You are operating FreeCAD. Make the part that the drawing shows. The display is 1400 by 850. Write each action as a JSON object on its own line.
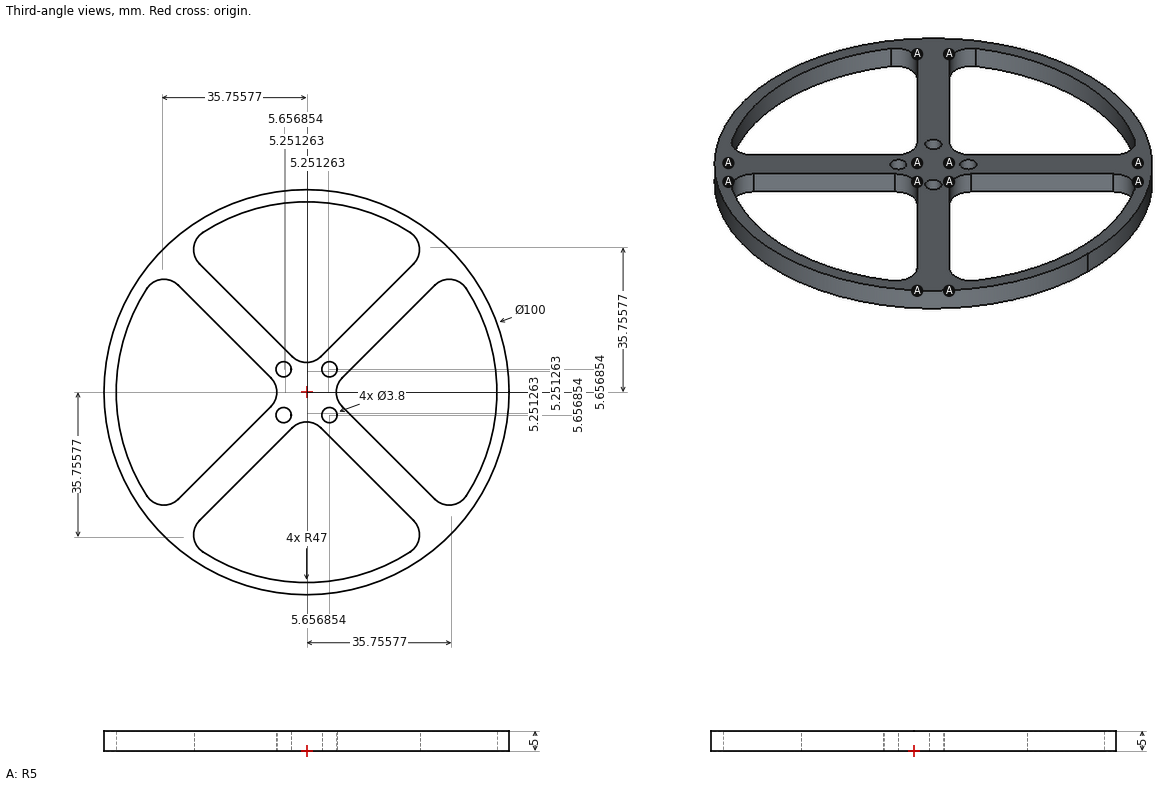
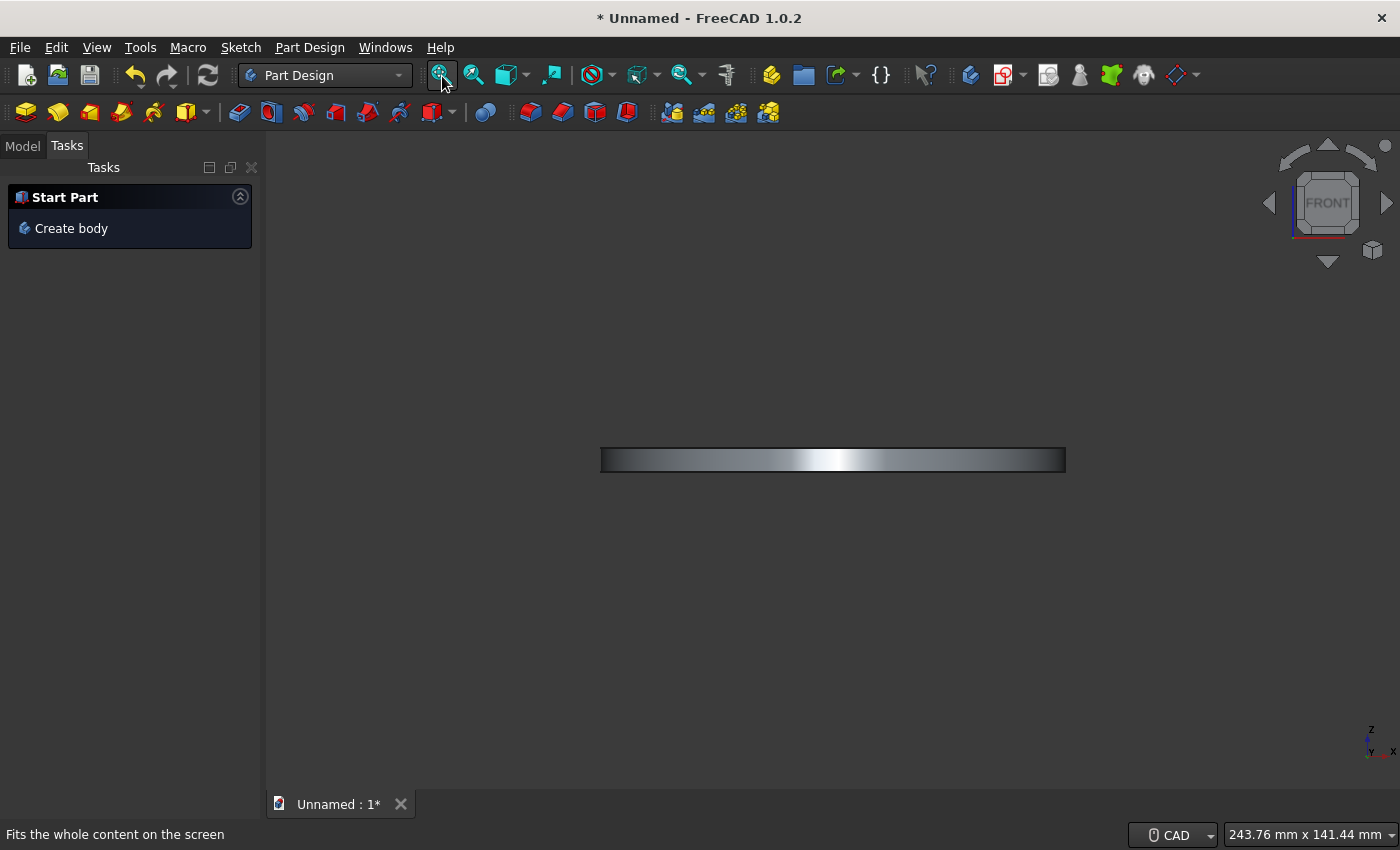
{"action": "left_click", "coordinate": [442, 76]}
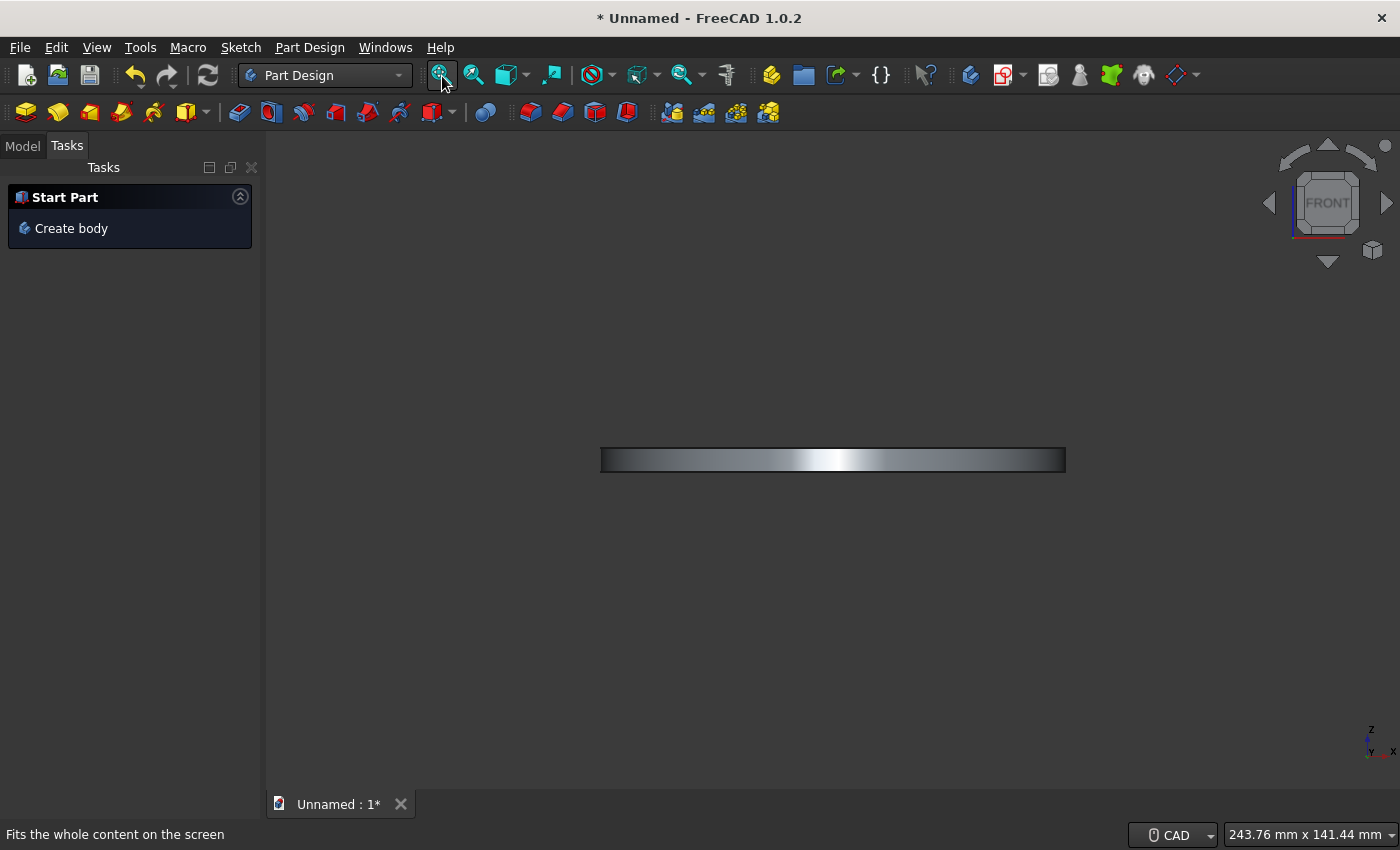
{"action": "key", "text": "3"}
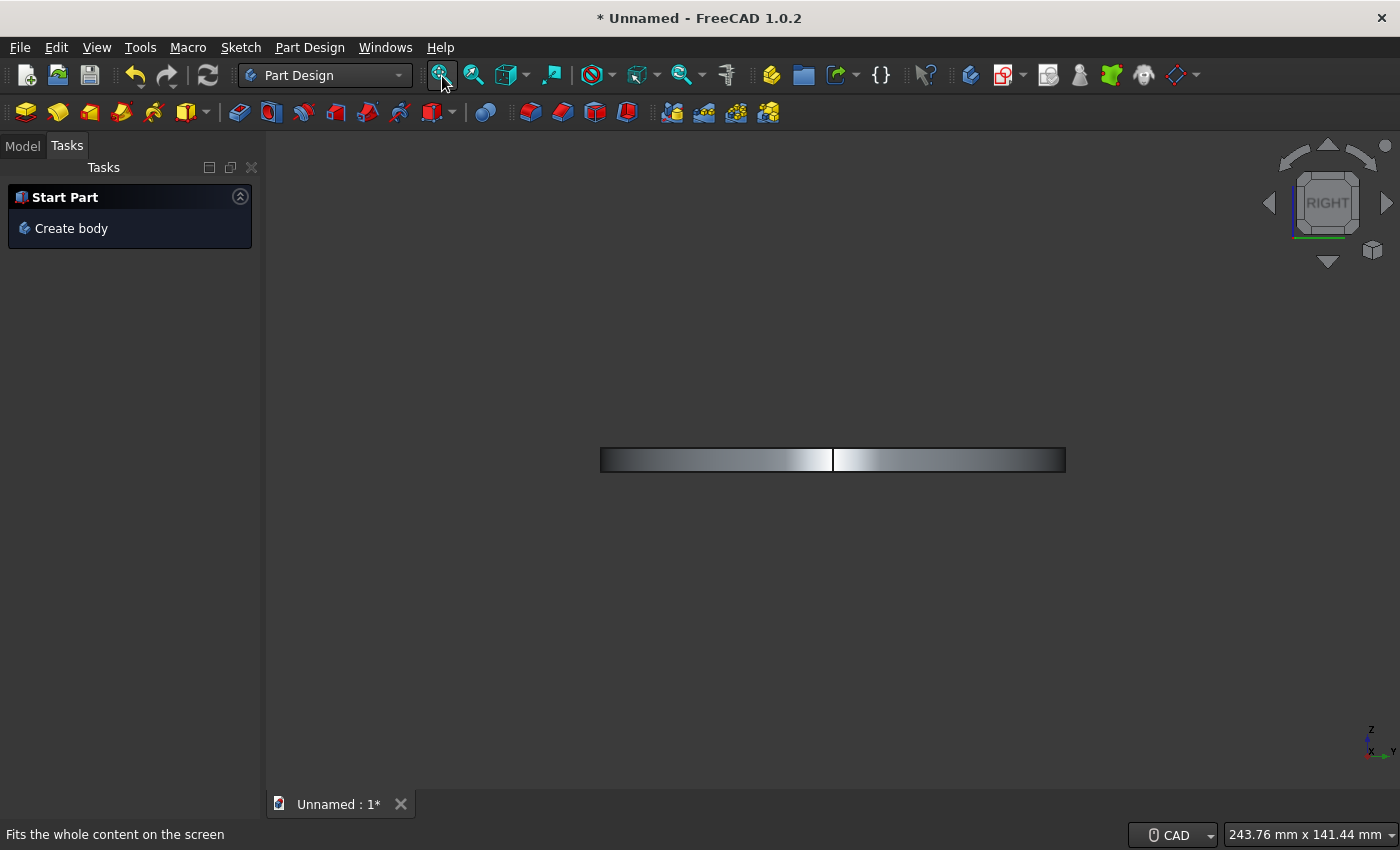
{"action": "left_click", "coordinate": [442, 76]}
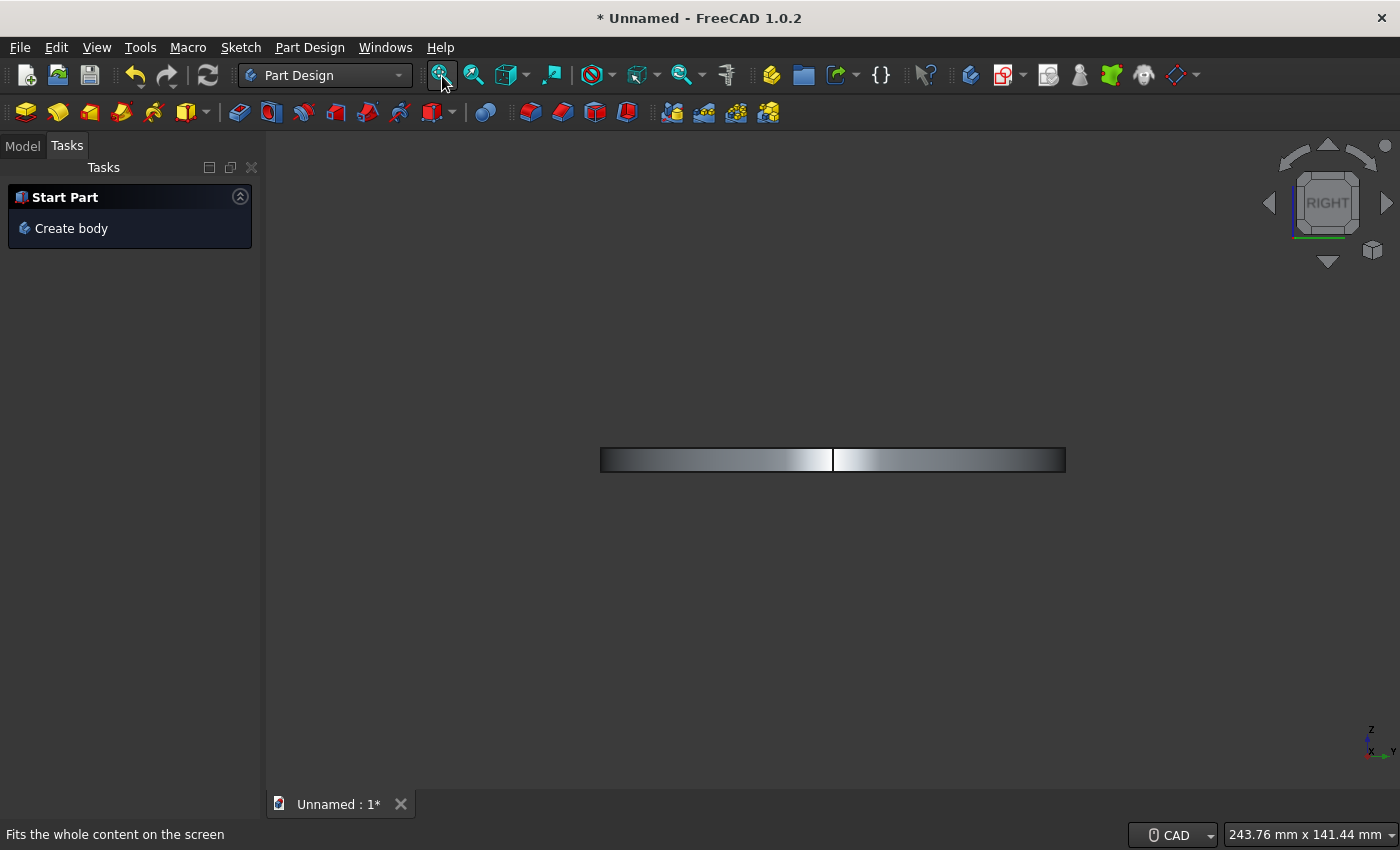
{"action": "key", "text": "5"}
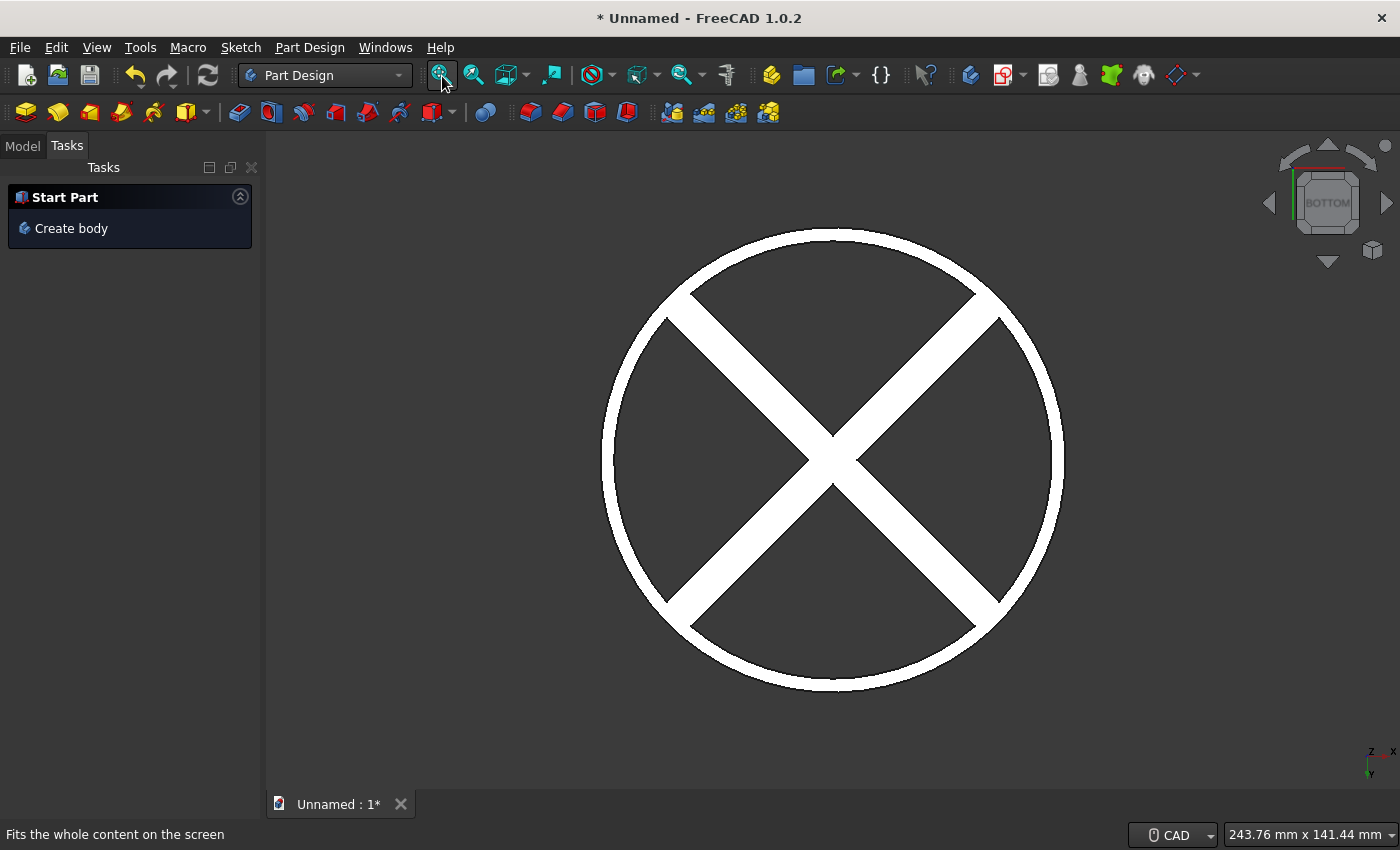
{"action": "key", "text": "4"}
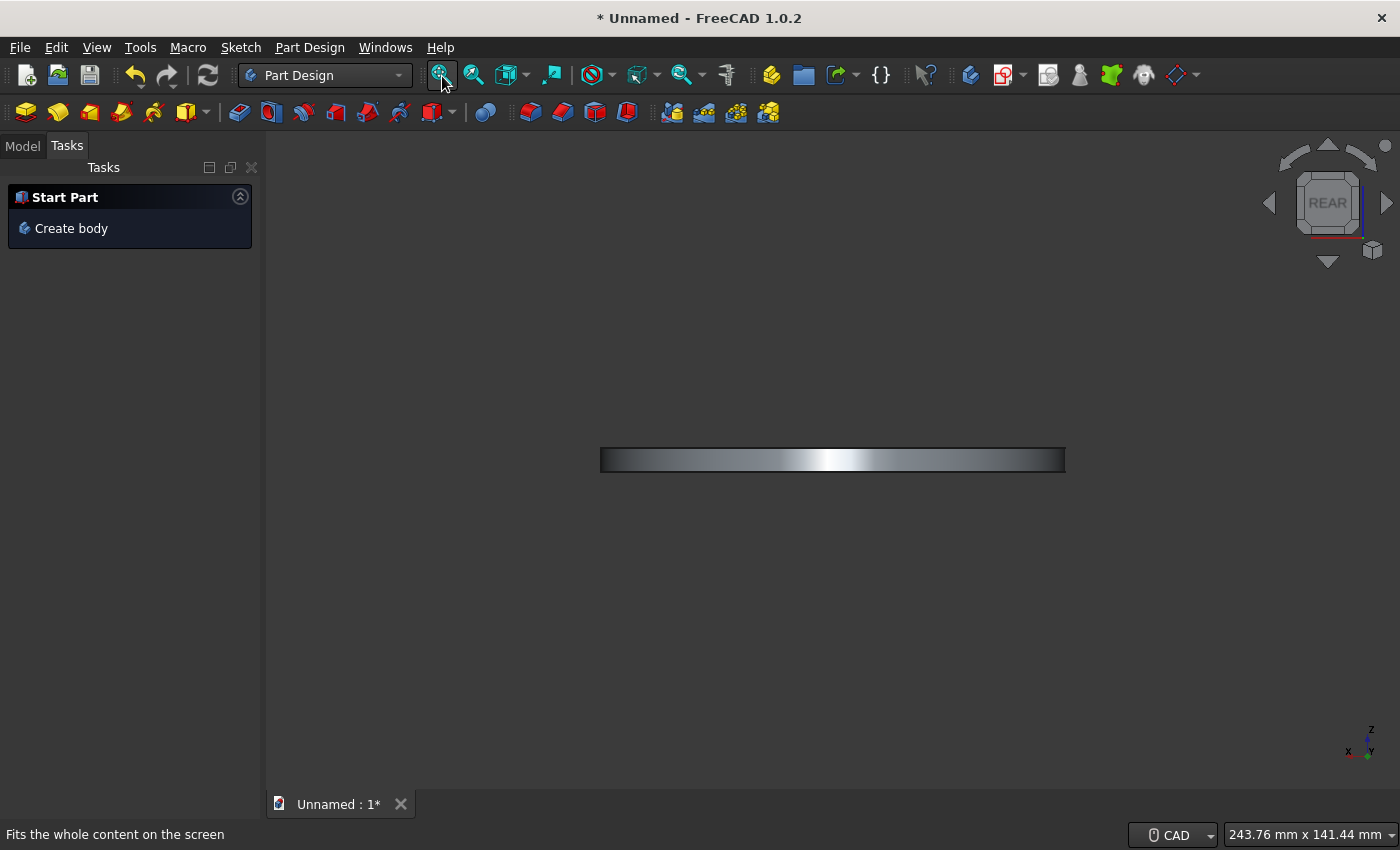
{"action": "left_click", "coordinate": [442, 76]}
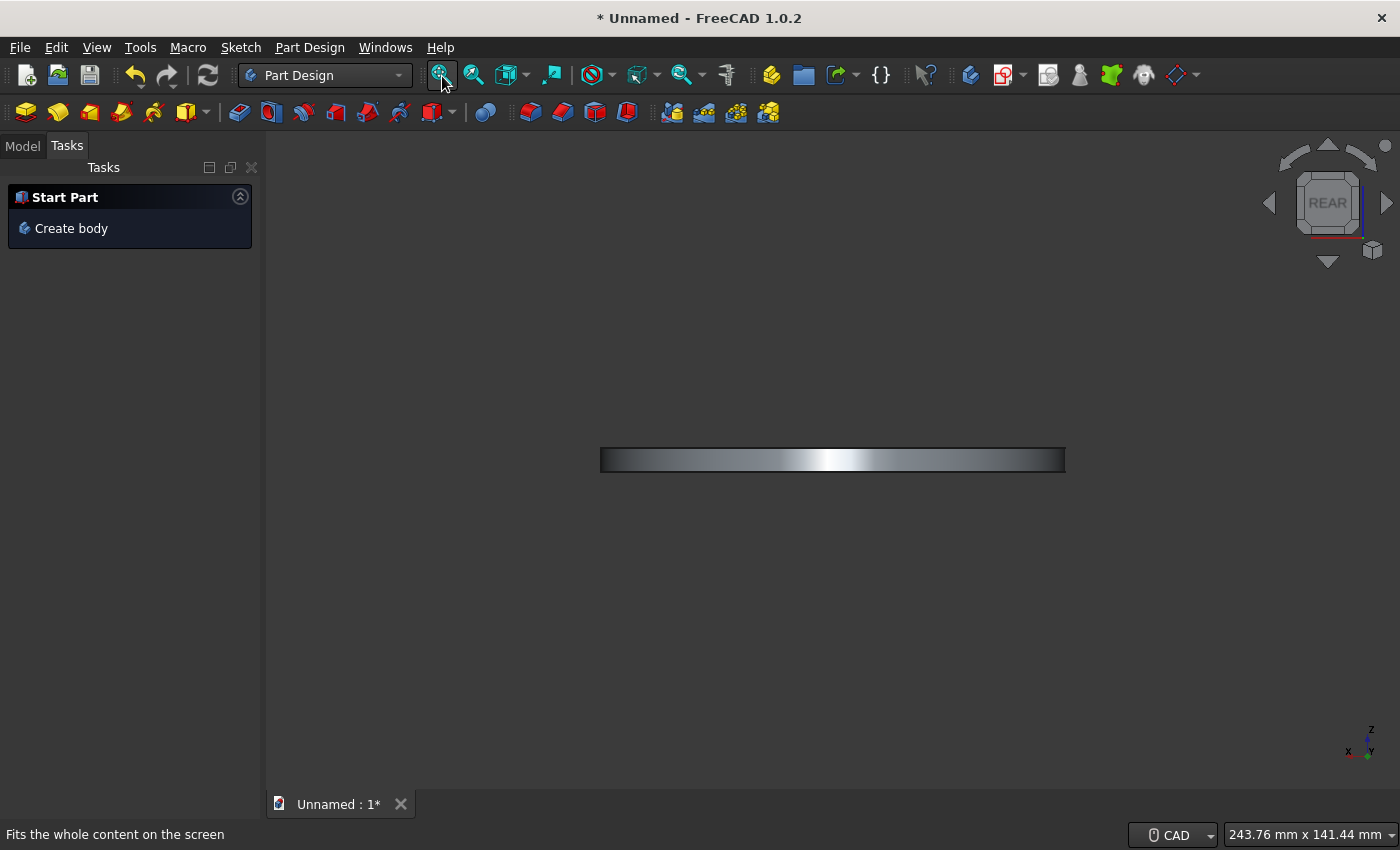
{"action": "key", "text": "6"}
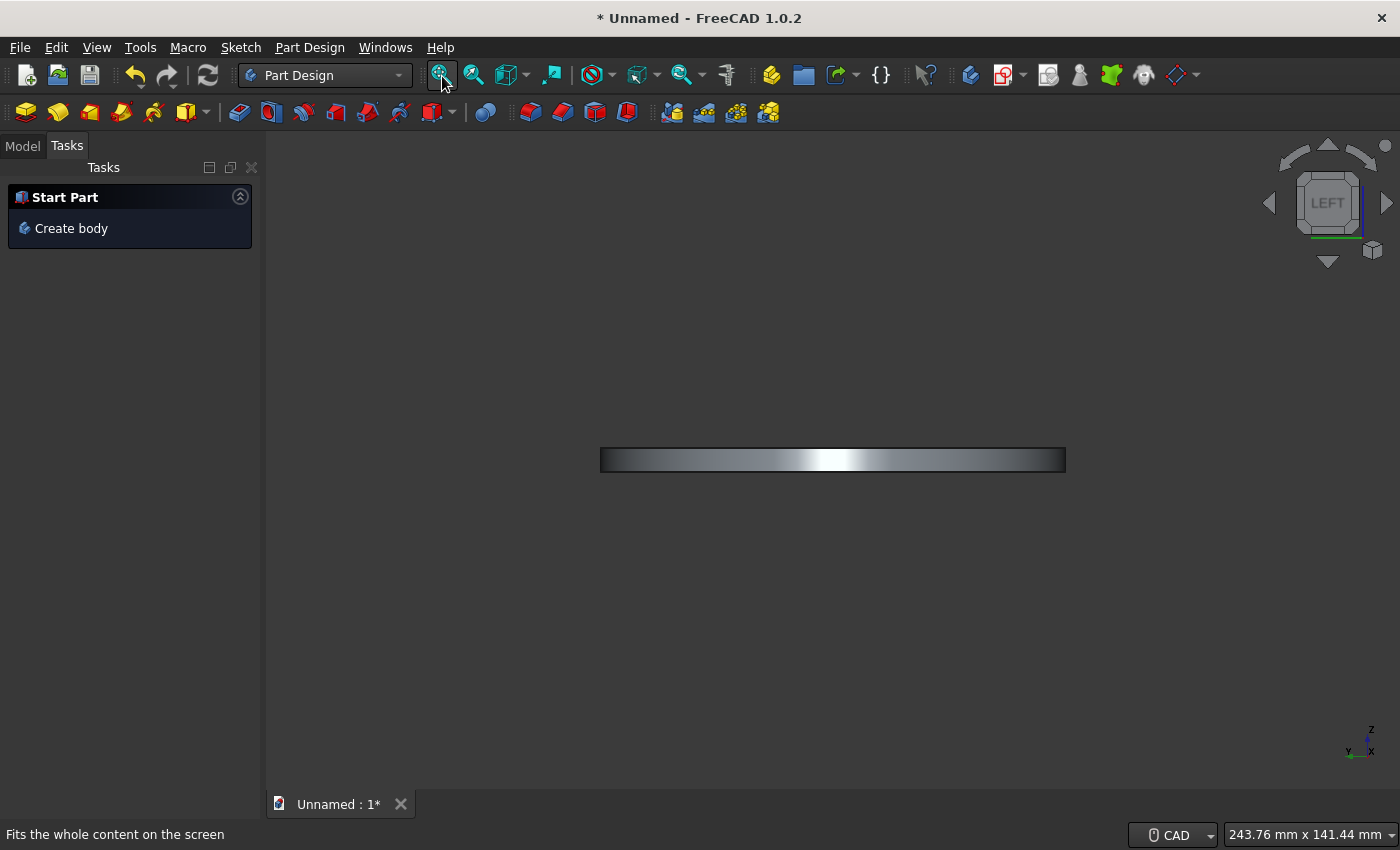
{"action": "left_click", "coordinate": [442, 76]}